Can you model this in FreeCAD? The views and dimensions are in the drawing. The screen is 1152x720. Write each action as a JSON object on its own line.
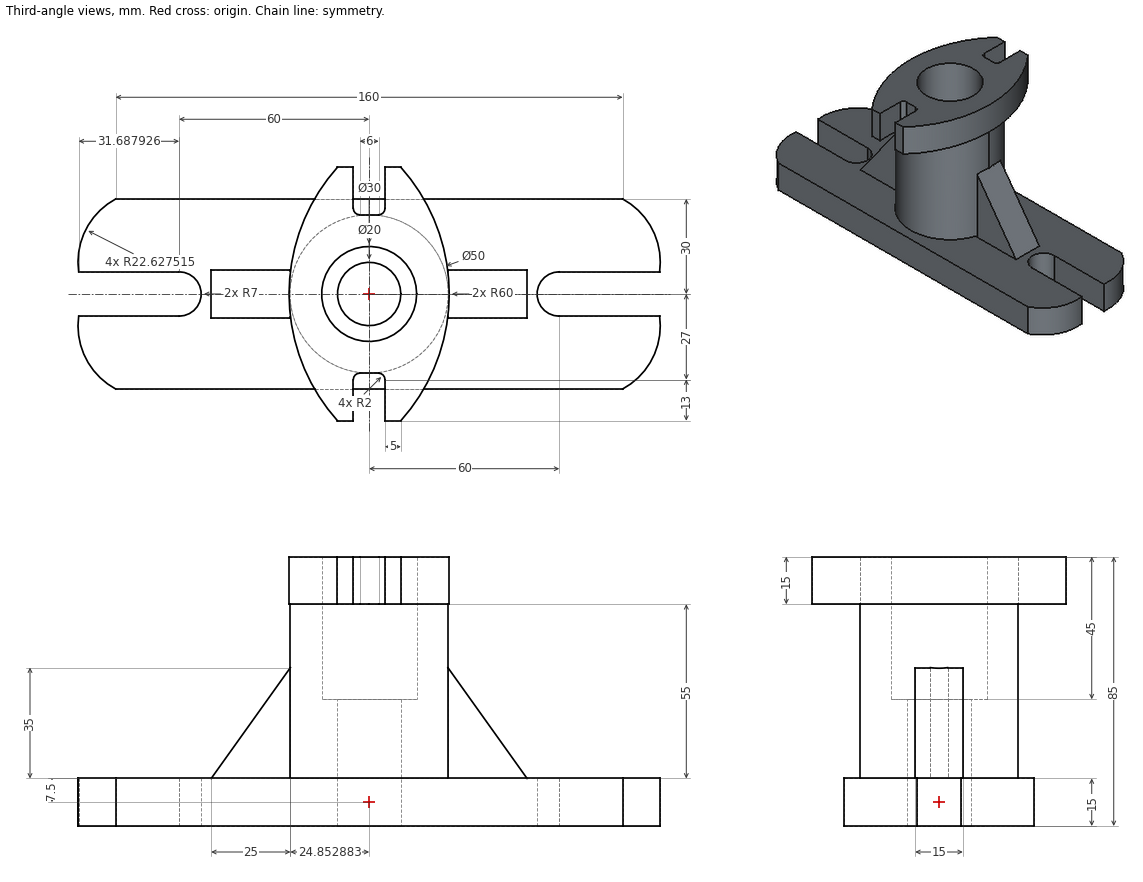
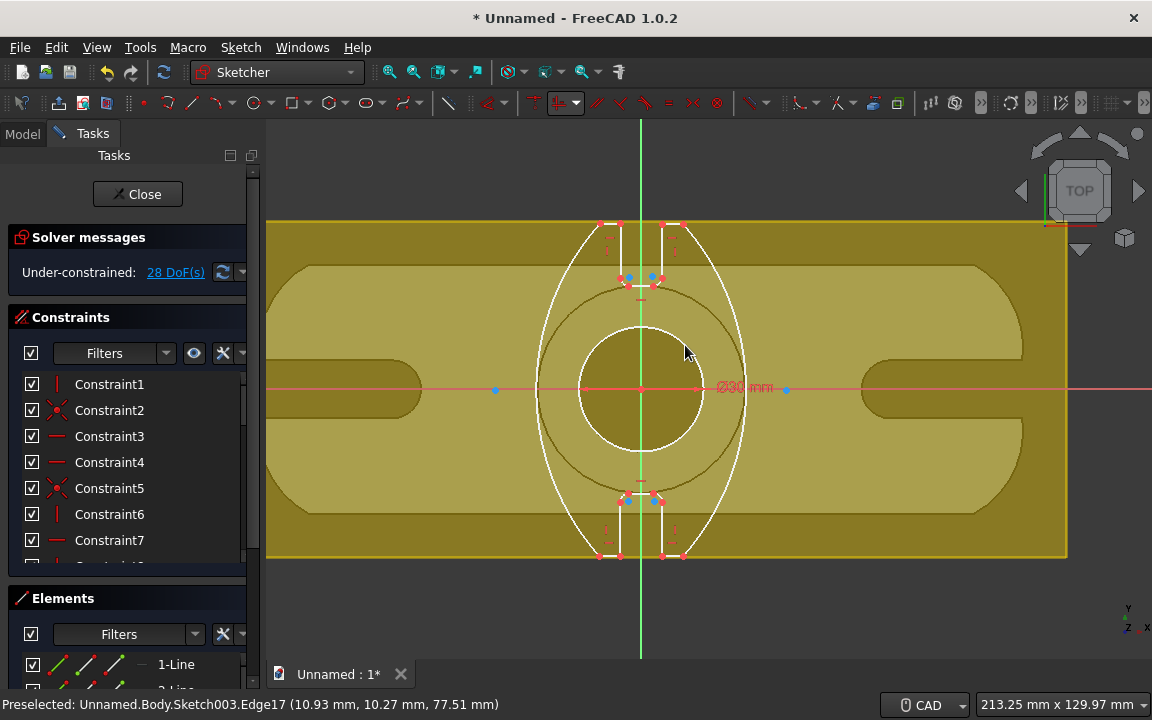
{"action": "left_click", "coordinate": [662, 519]}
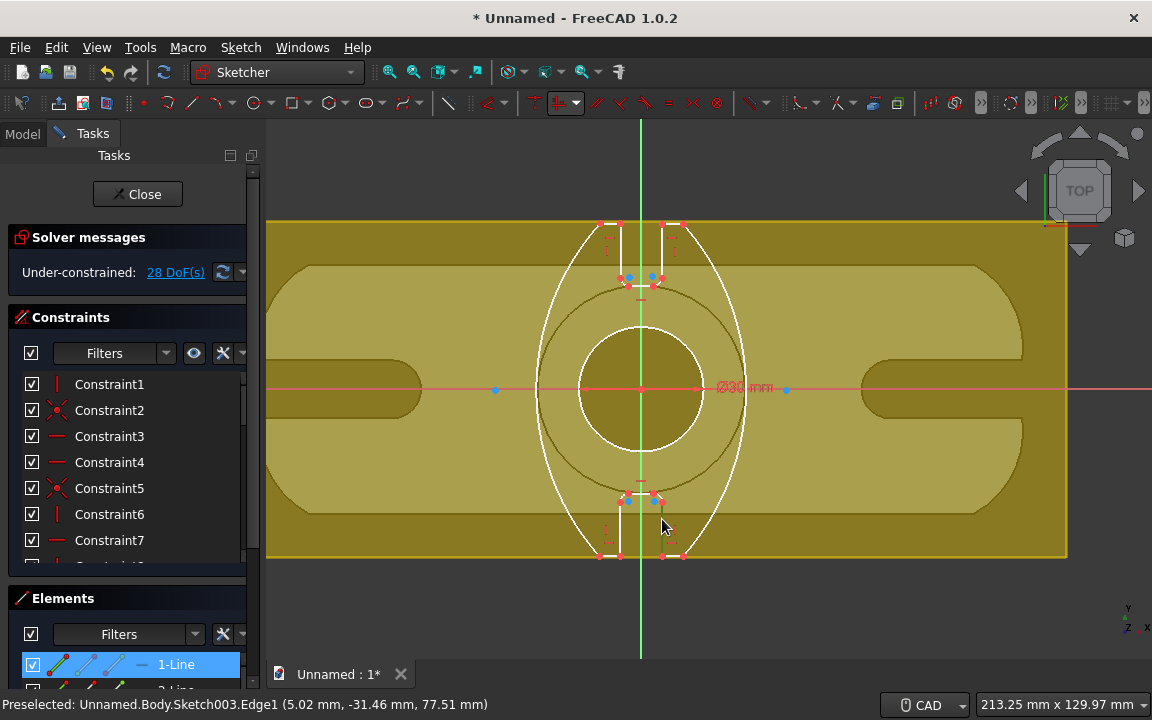
{"action": "scroll", "coordinate": [660, 496], "scroll_direction": "up", "scroll_amount": 4}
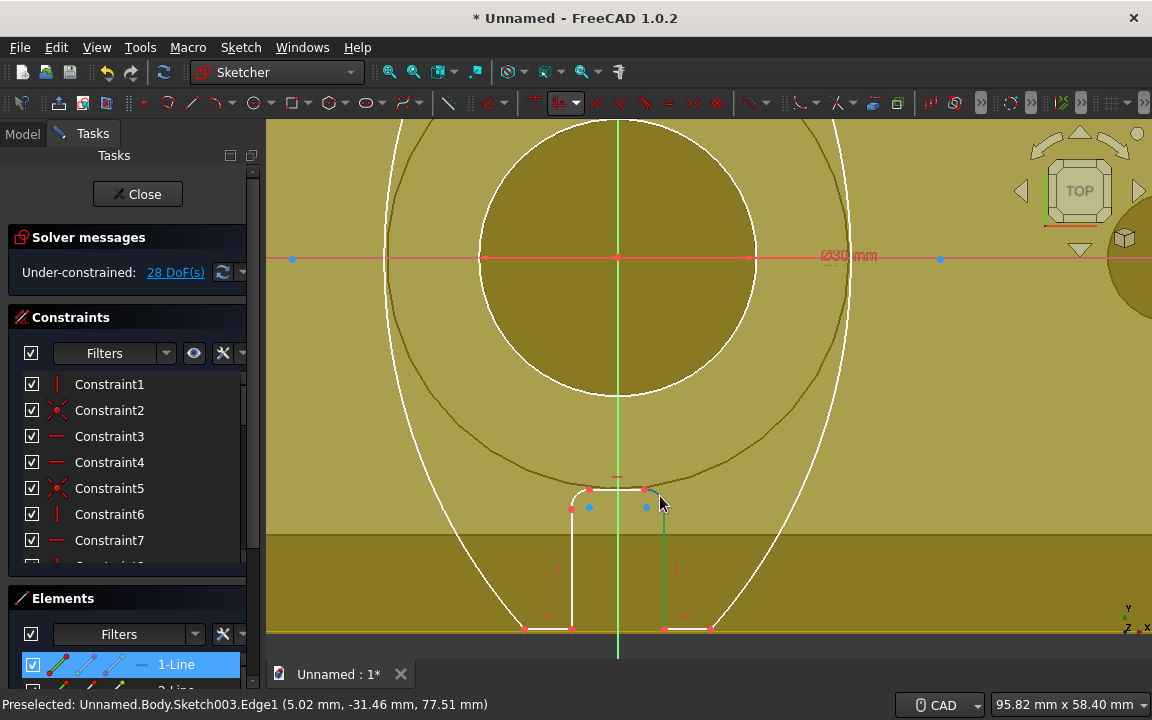
{"action": "left_click", "coordinate": [659, 495]}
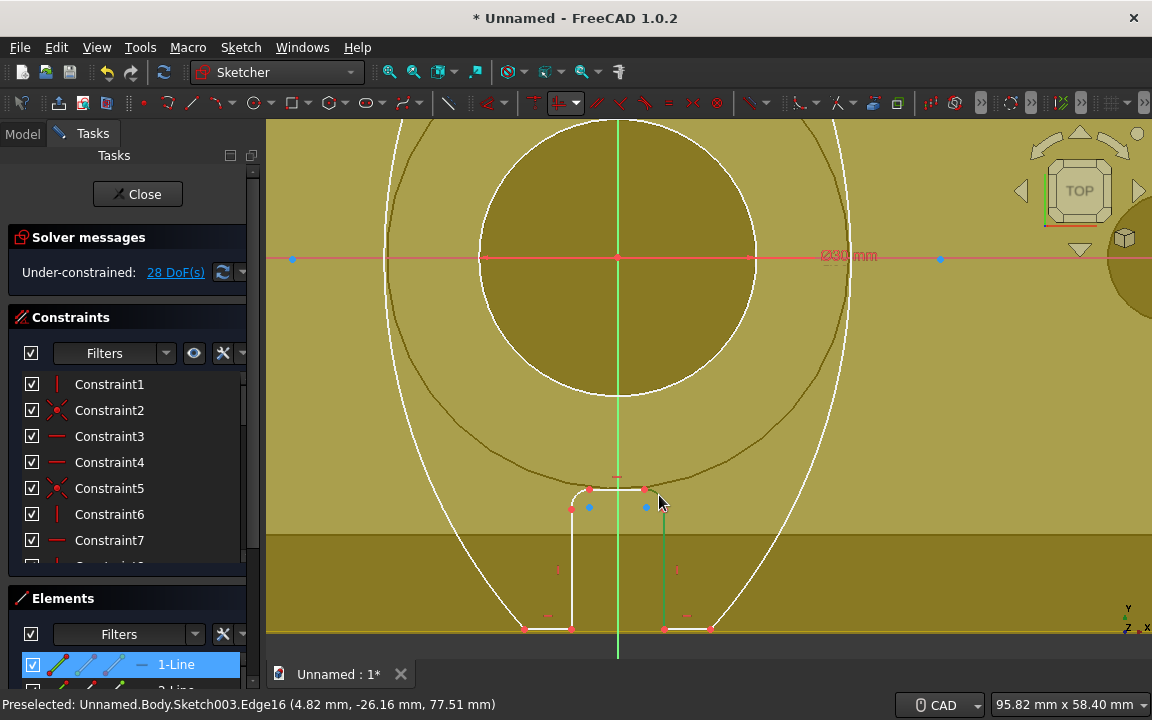
{"action": "key", "text": "t"}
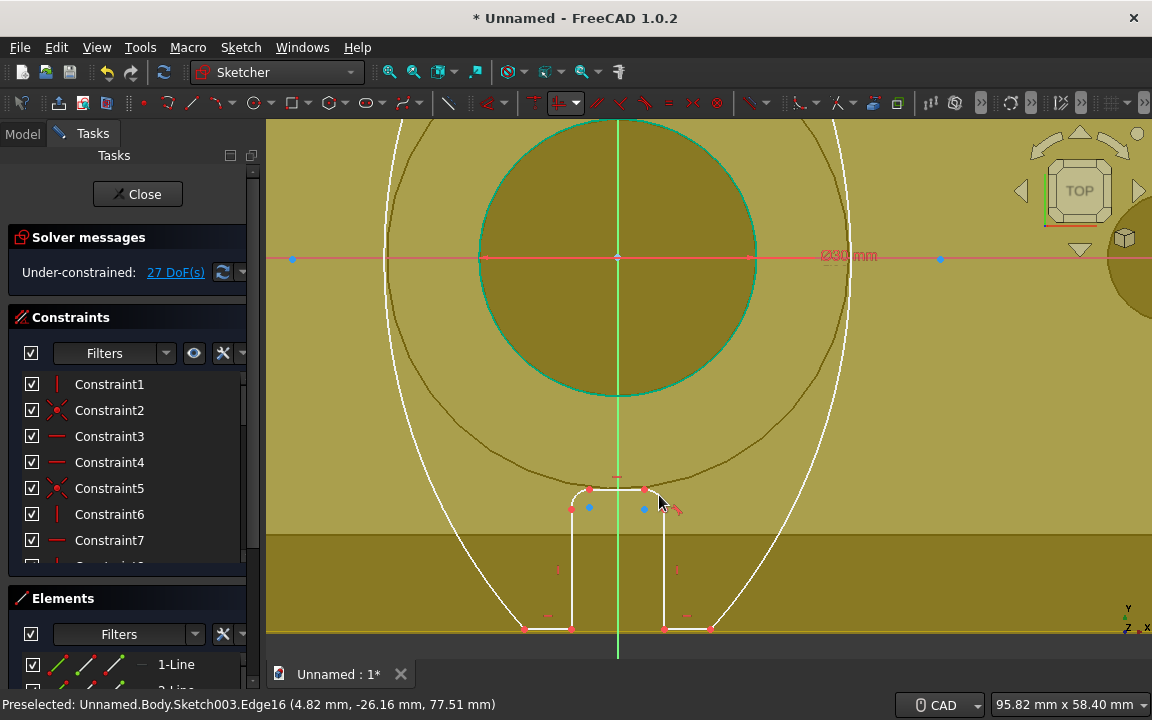
{"action": "scroll", "coordinate": [659, 496], "scroll_direction": "down", "scroll_amount": 4}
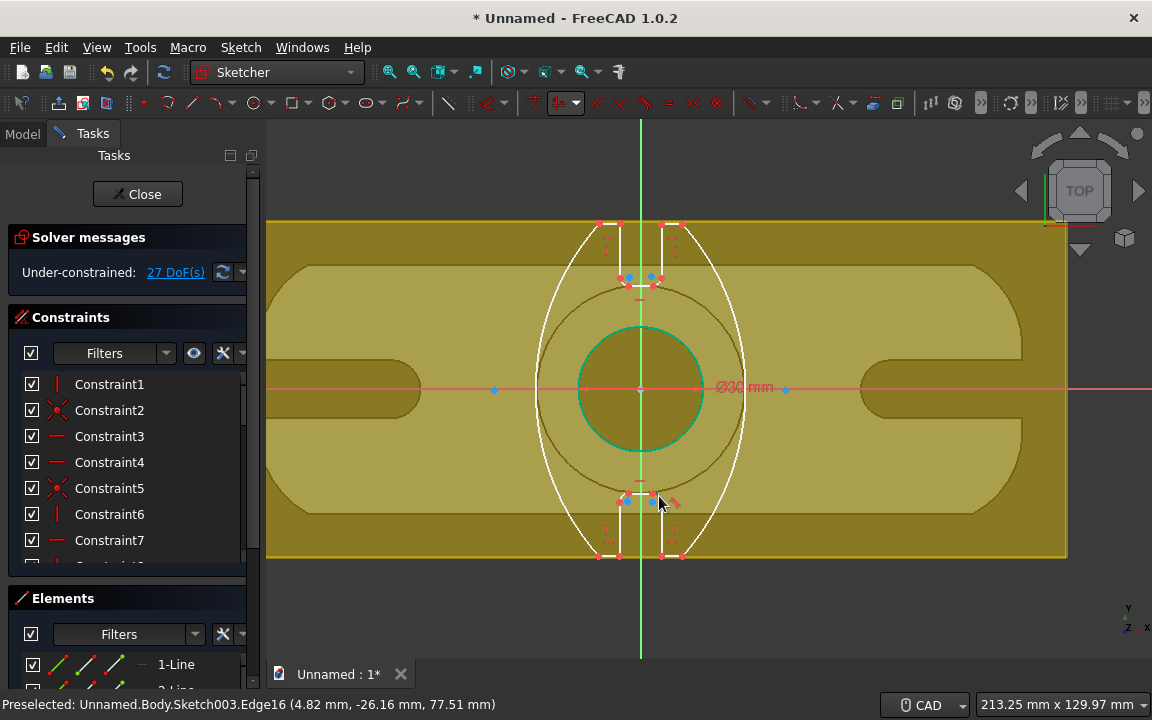
{"action": "left_click", "coordinate": [662, 241]}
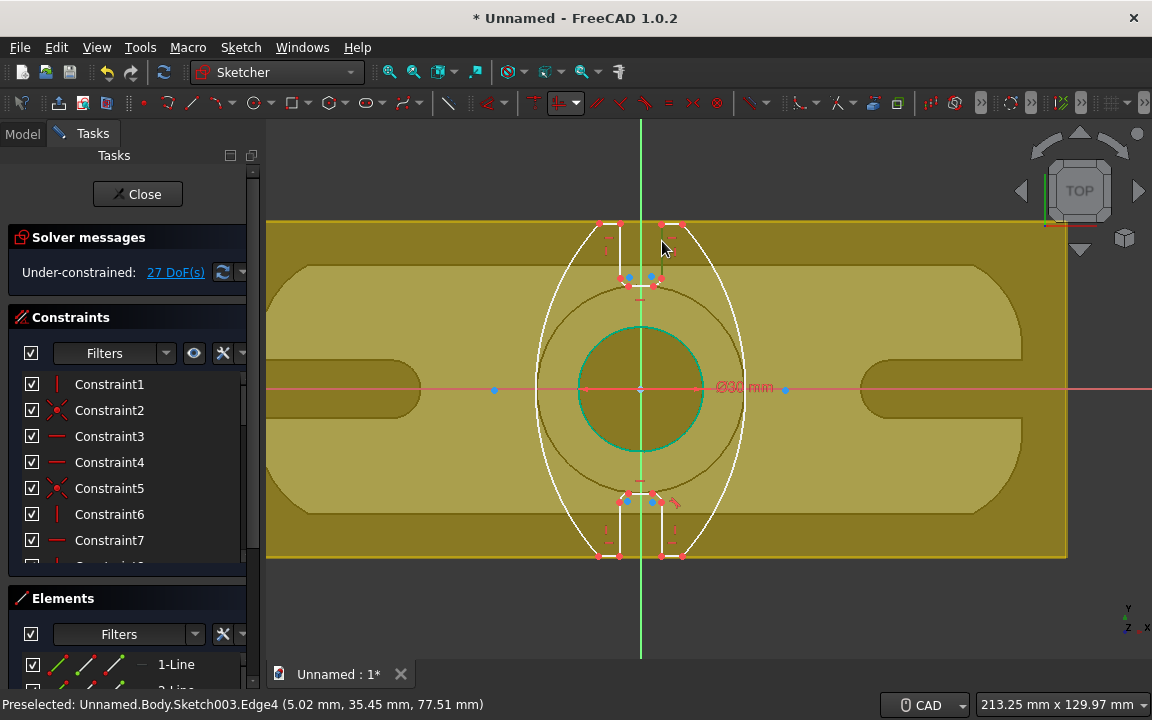
{"action": "scroll", "coordinate": [659, 284], "scroll_direction": "up", "scroll_amount": 5}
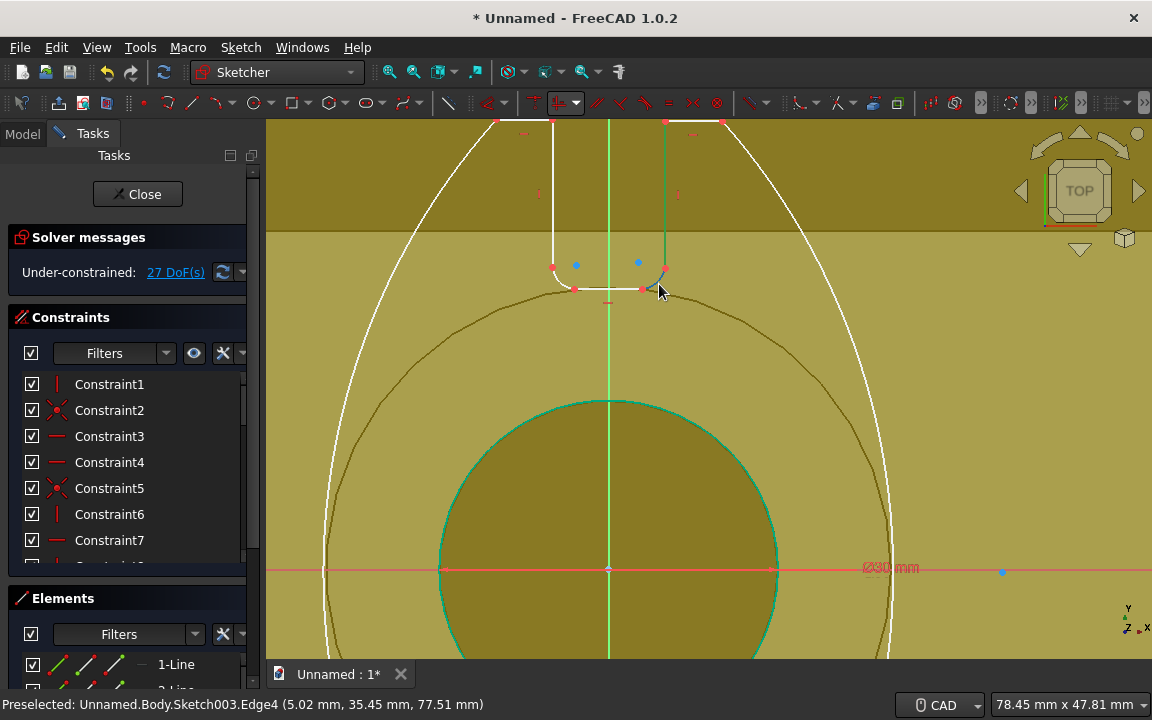
{"action": "left_click", "coordinate": [657, 282]}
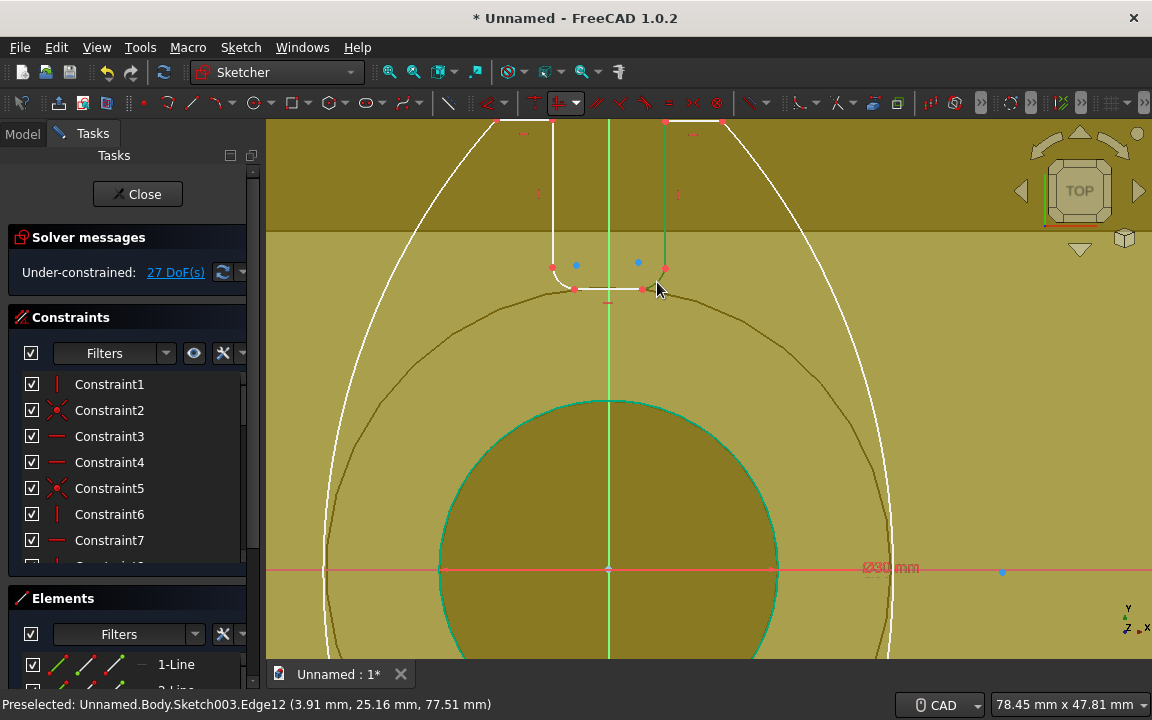
{"action": "key", "text": "t"}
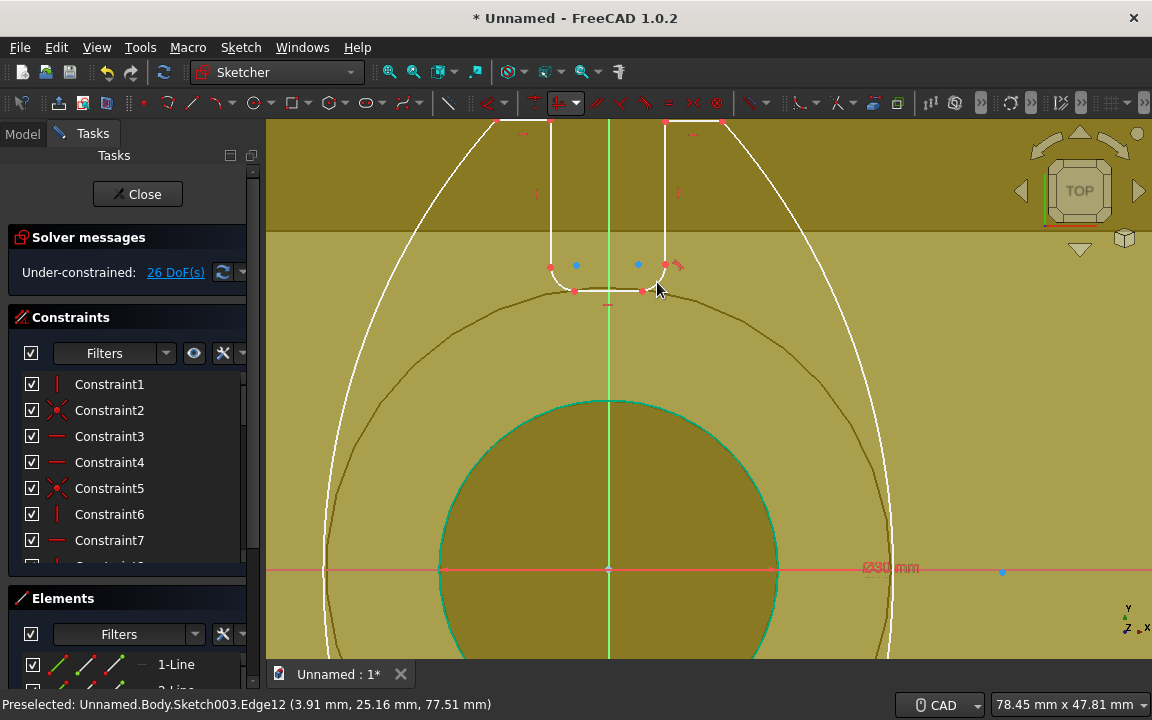
{"action": "left_click", "coordinate": [622, 291]}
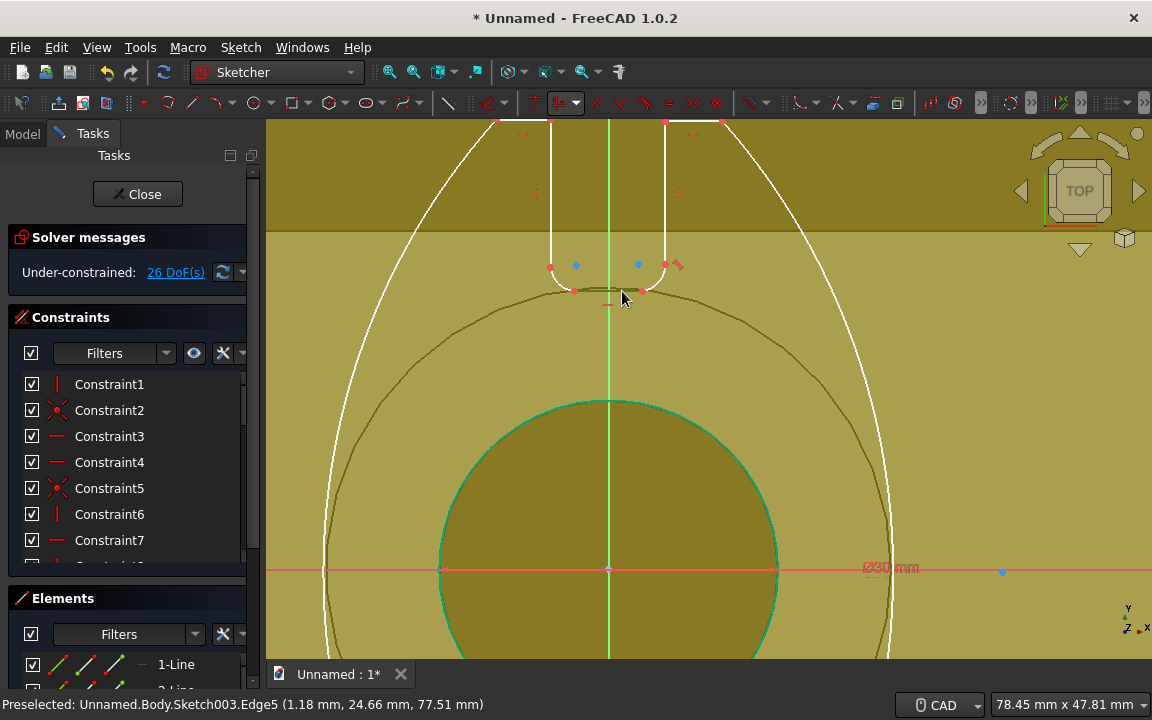
{"action": "left_click", "coordinate": [653, 287]}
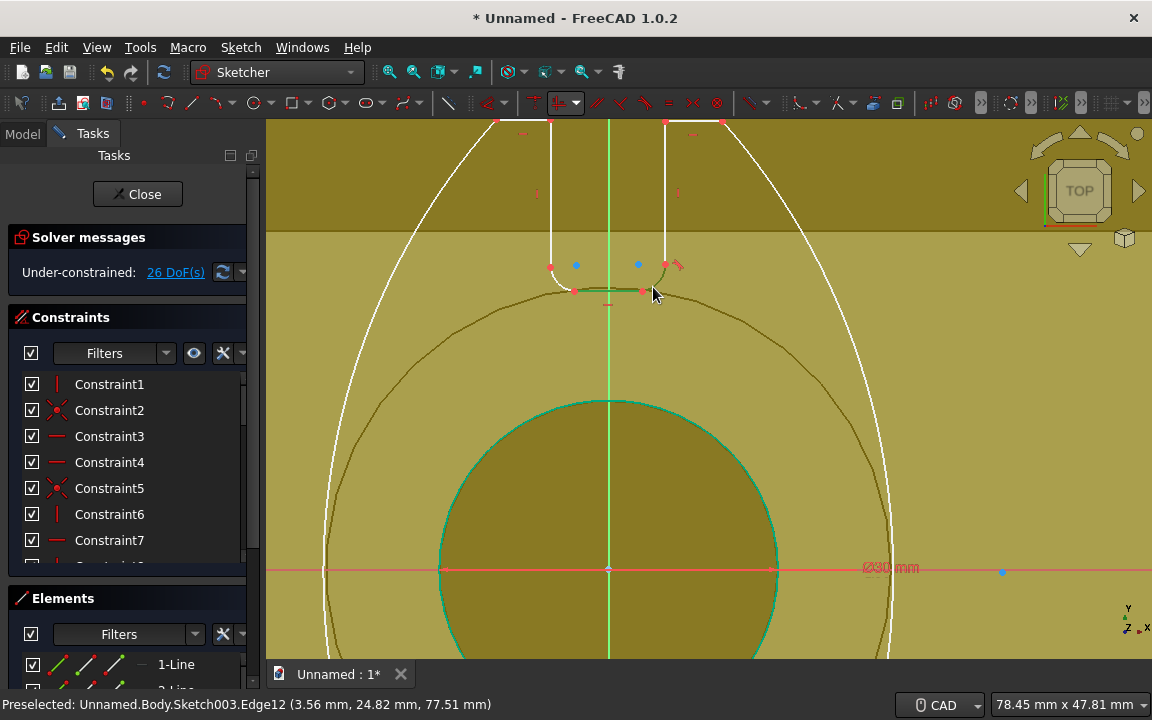
{"action": "key", "text": "t"}